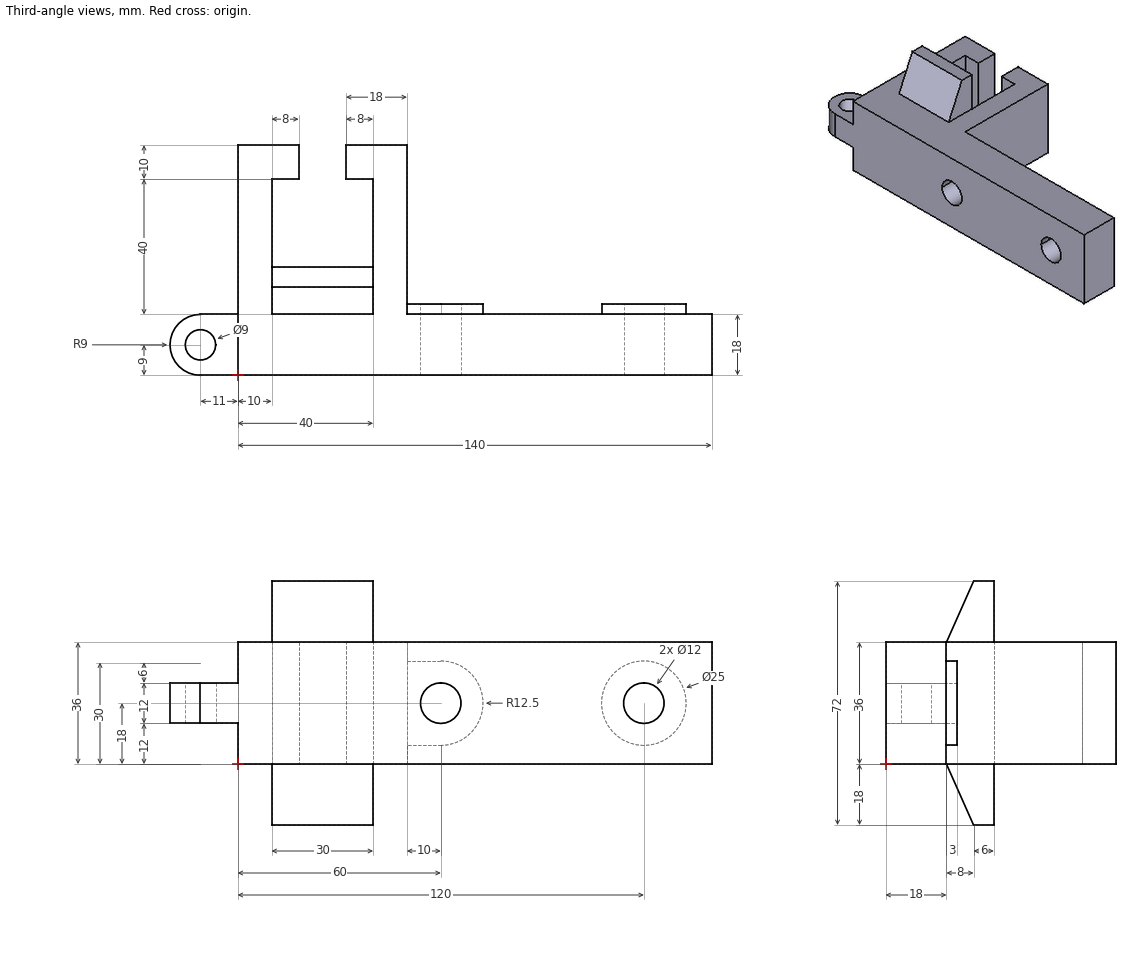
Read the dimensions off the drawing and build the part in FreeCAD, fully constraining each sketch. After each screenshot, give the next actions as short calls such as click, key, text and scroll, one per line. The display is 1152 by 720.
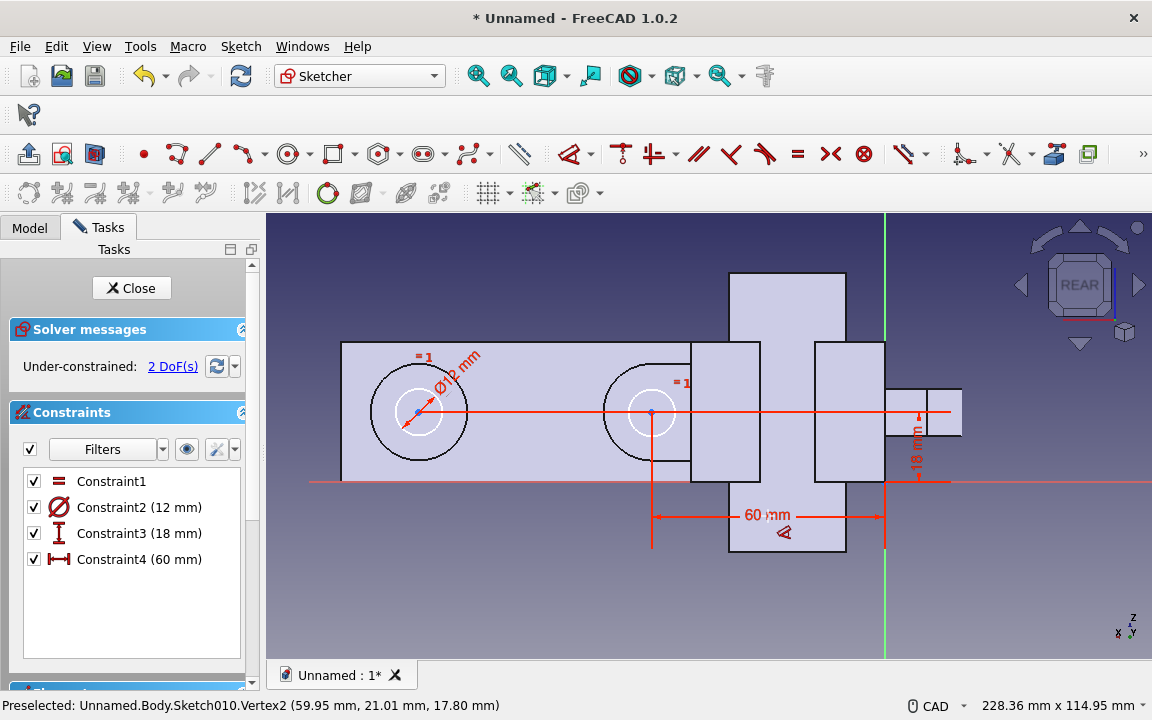
click(652, 413)
click(919, 423)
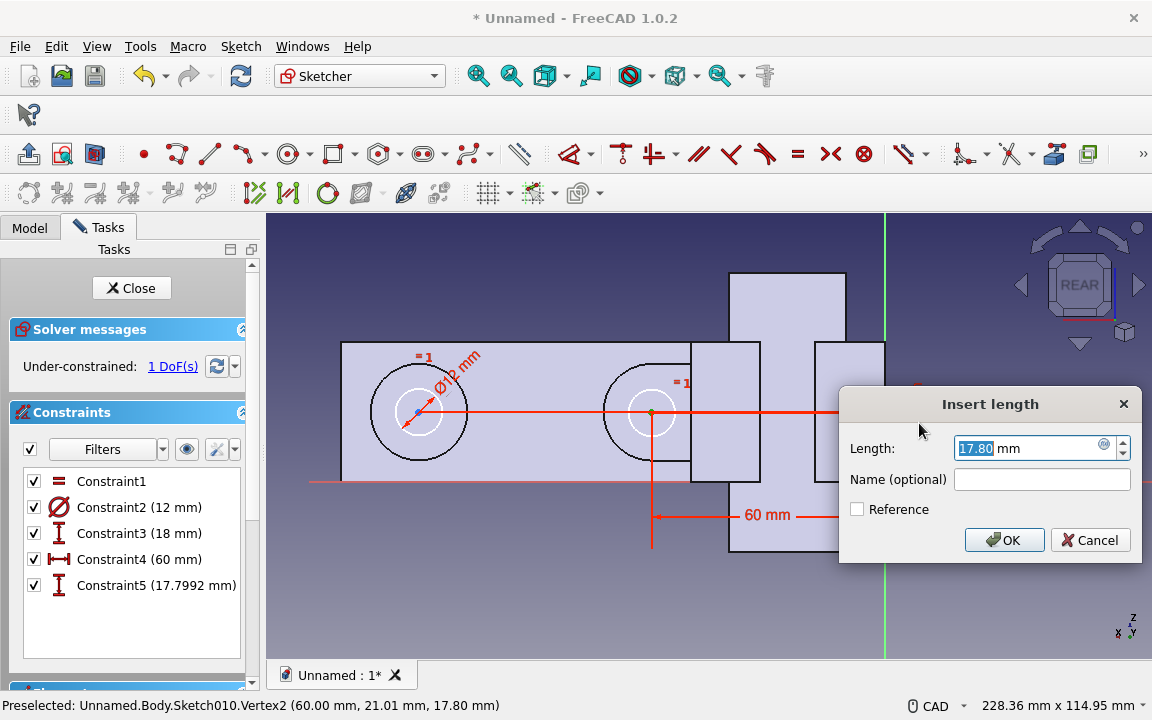
text(18)
key(Return)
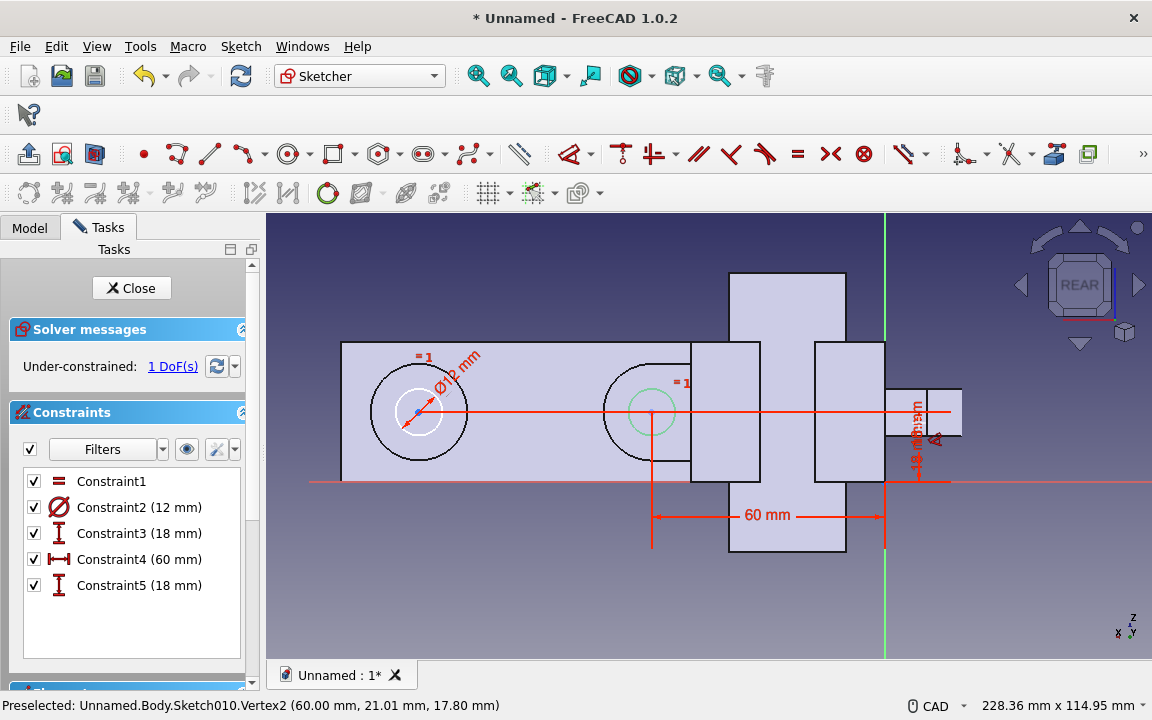
click(419, 412)
click(652, 516)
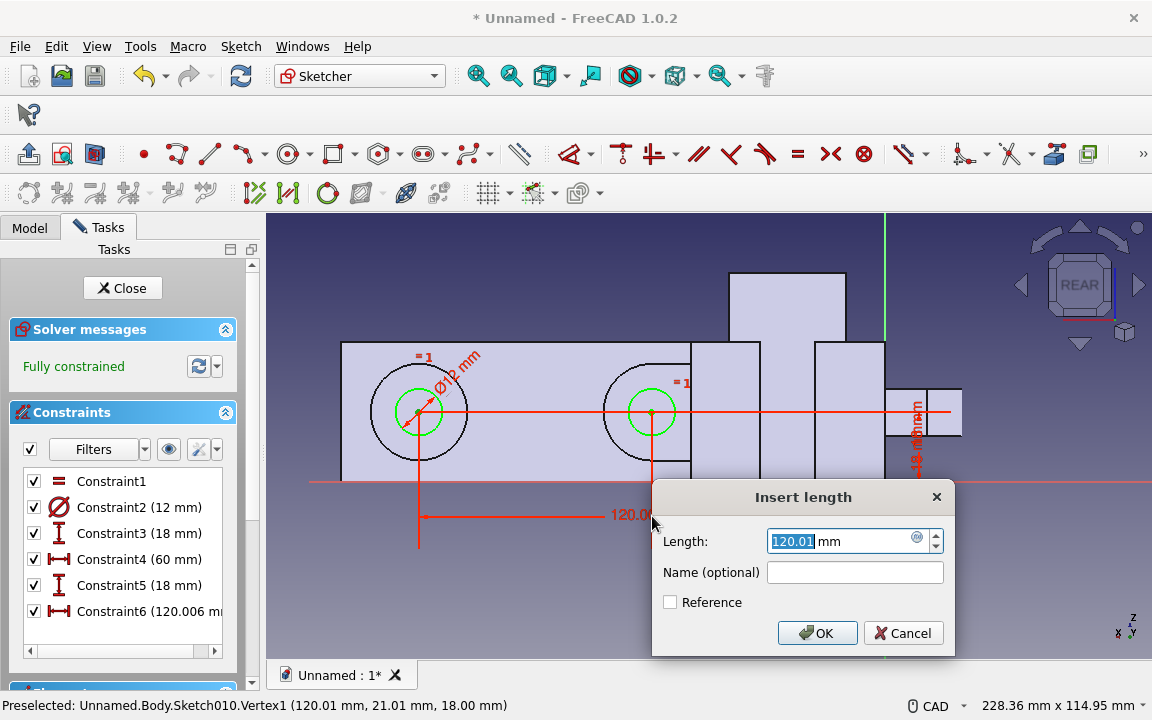
text(120)
key(Return)
key(Escape)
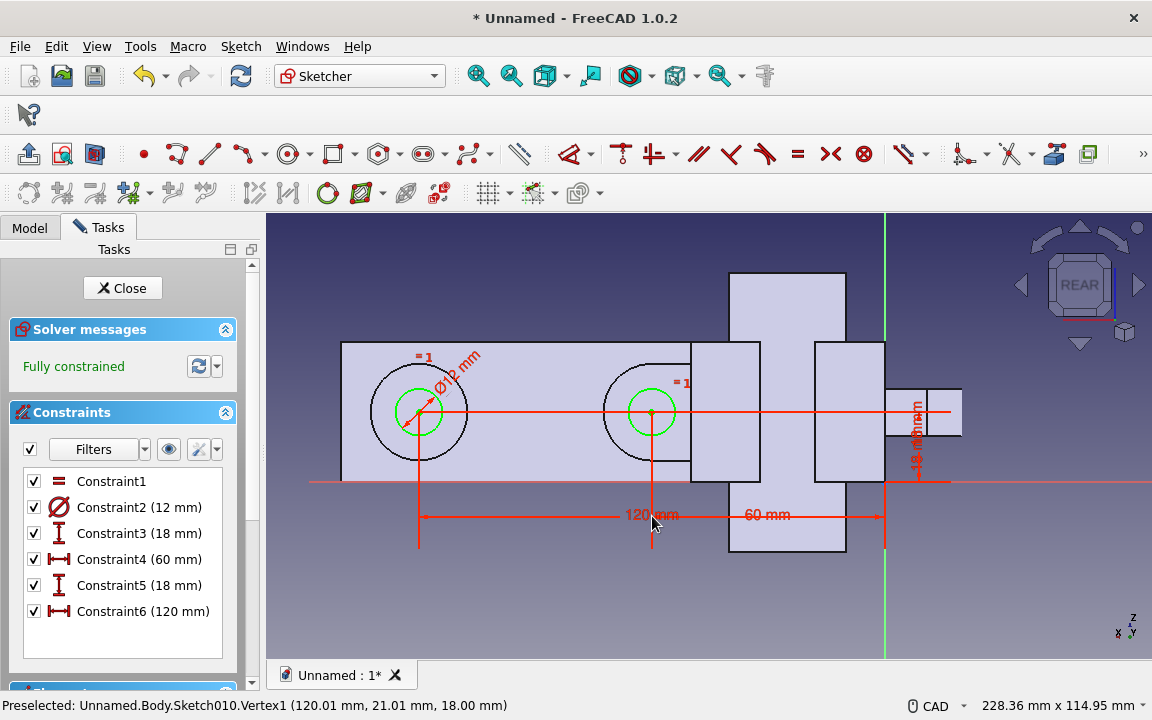
click(123, 288)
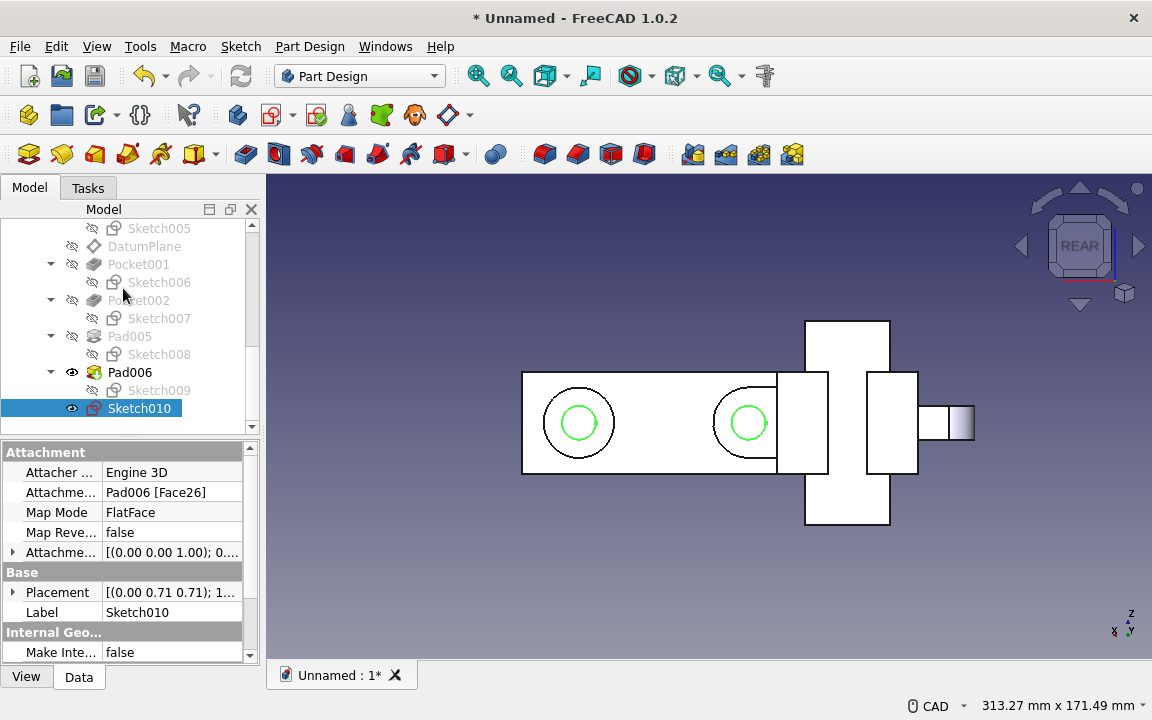
click(246, 154)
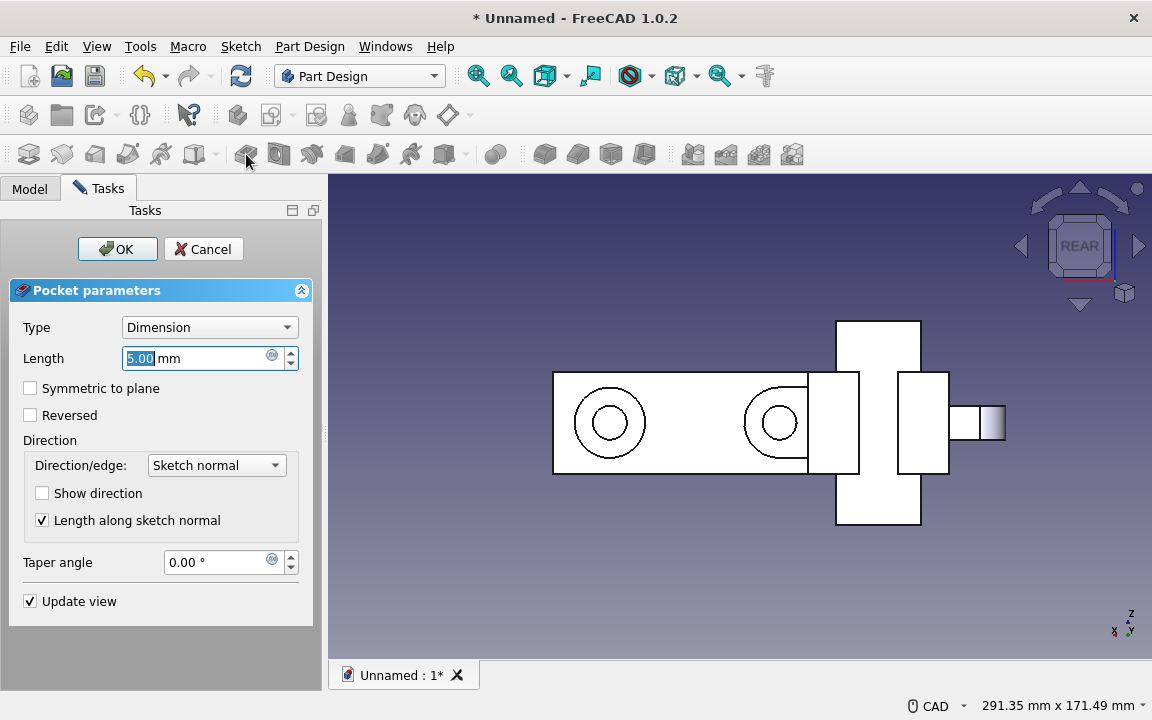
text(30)
key(Tab)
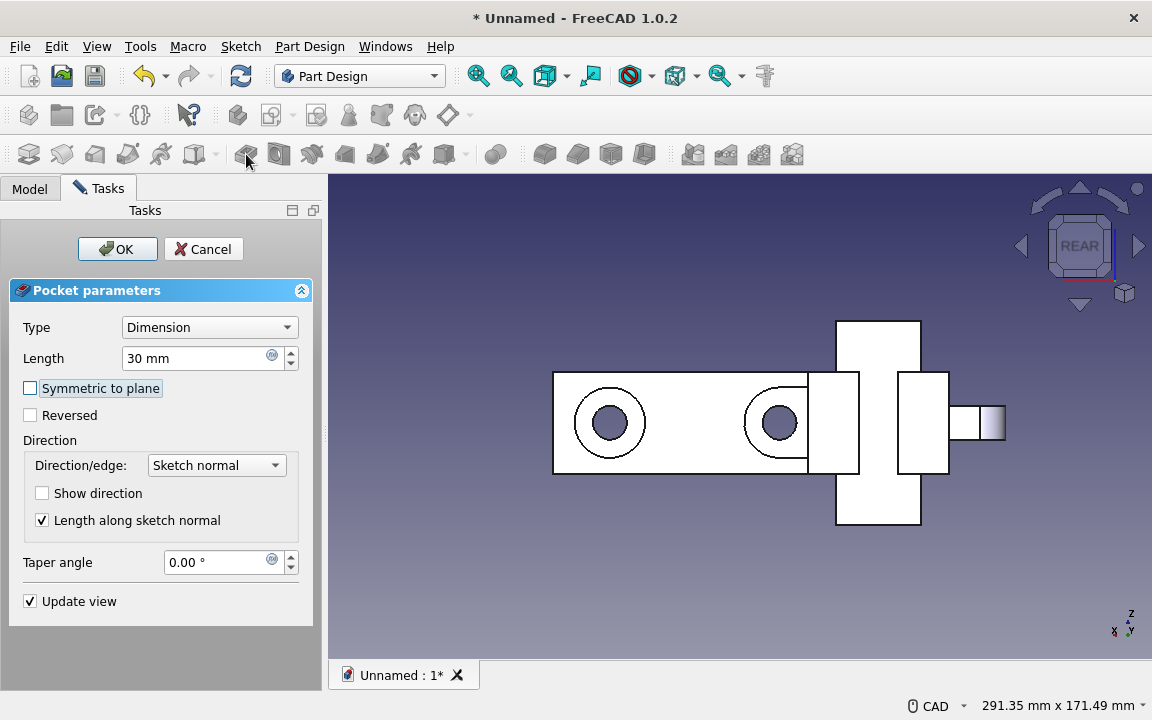
click(118, 249)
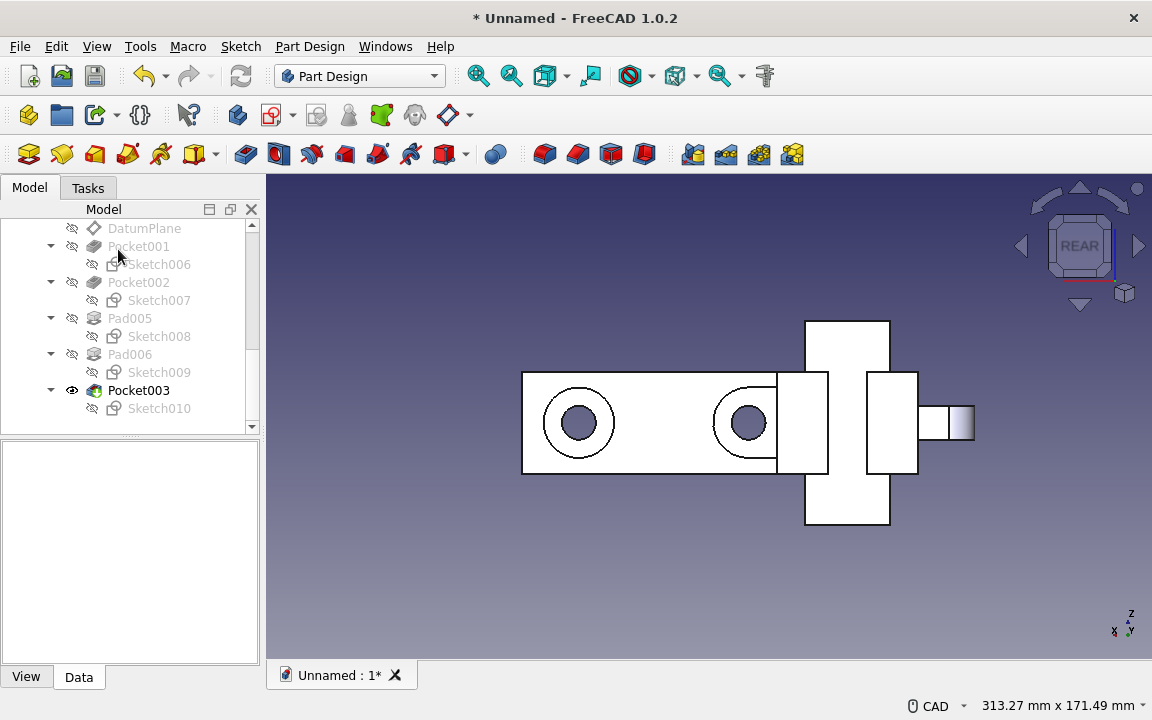
key(0)